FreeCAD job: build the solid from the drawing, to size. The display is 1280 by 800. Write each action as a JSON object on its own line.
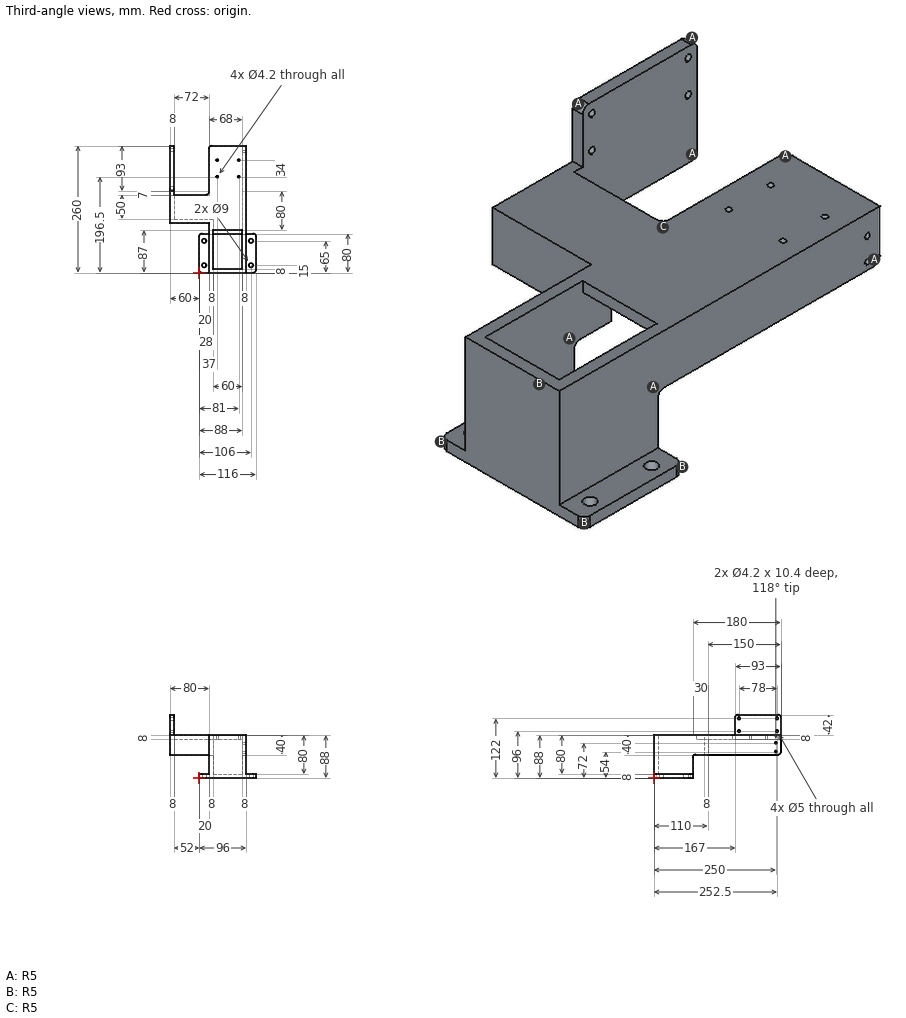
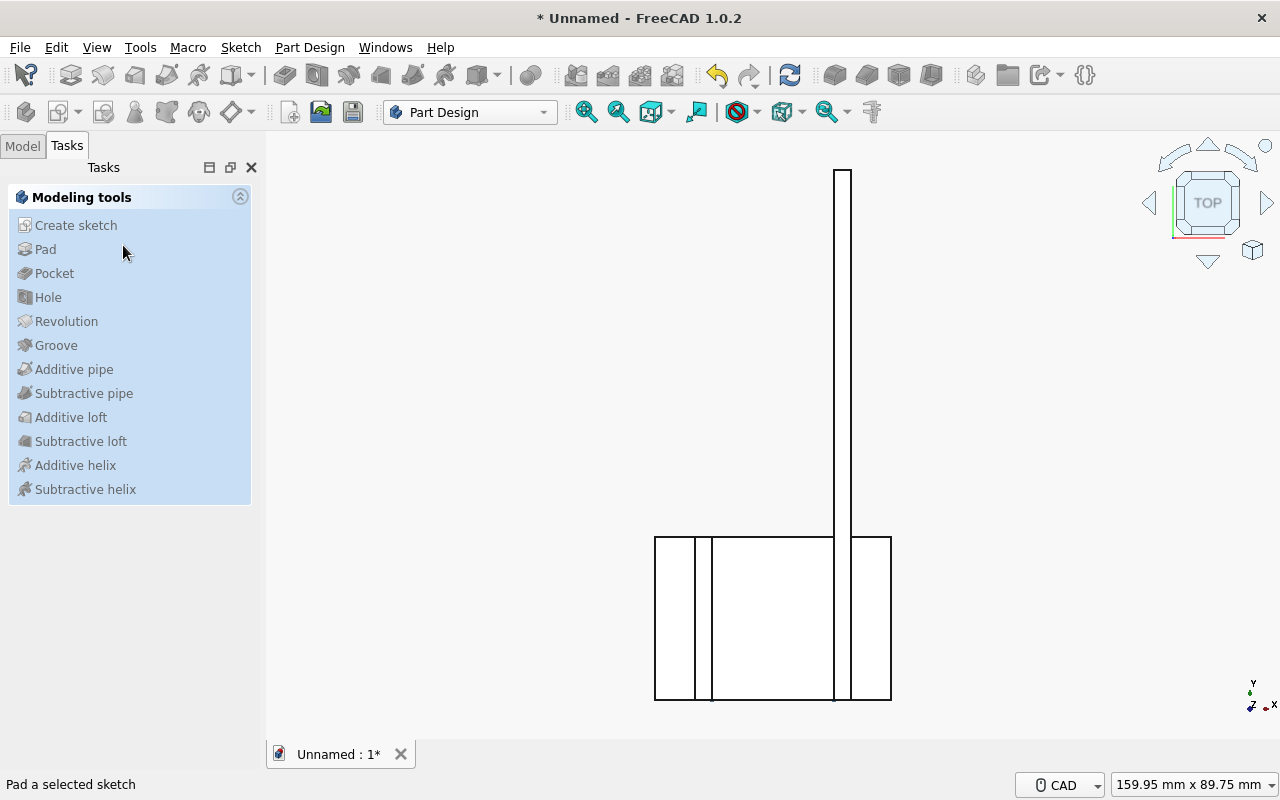
{"action": "left_click", "coordinate": [72, 76]}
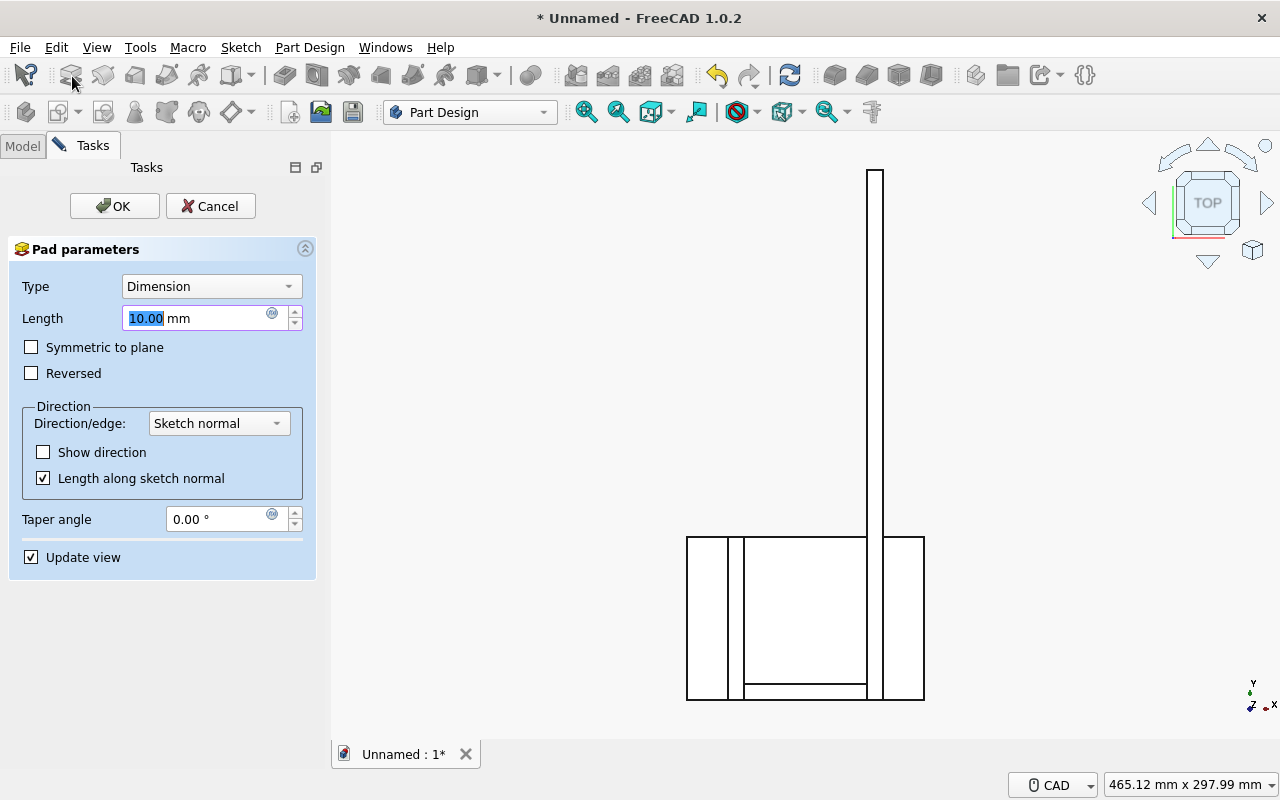
{"action": "type", "text": "80"}
{"action": "key", "text": "Tab"}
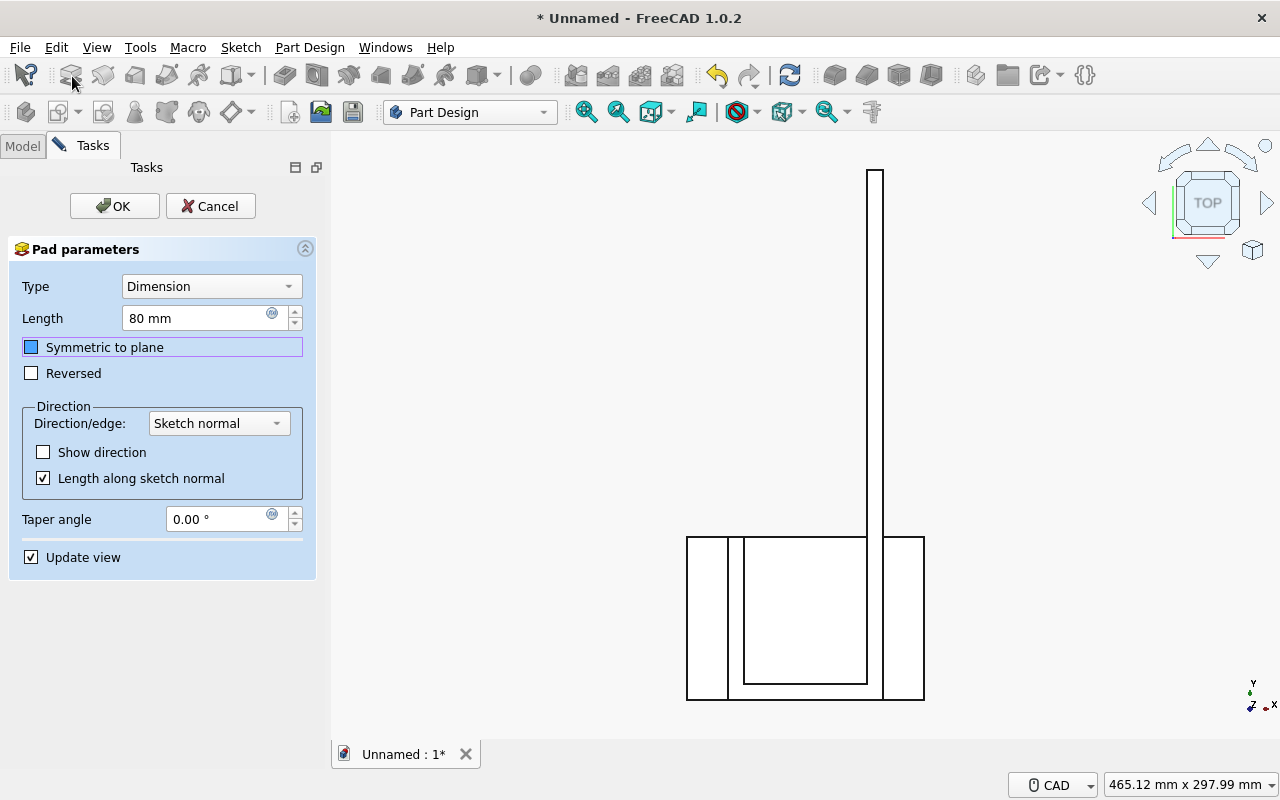
{"action": "left_click", "coordinate": [115, 206]}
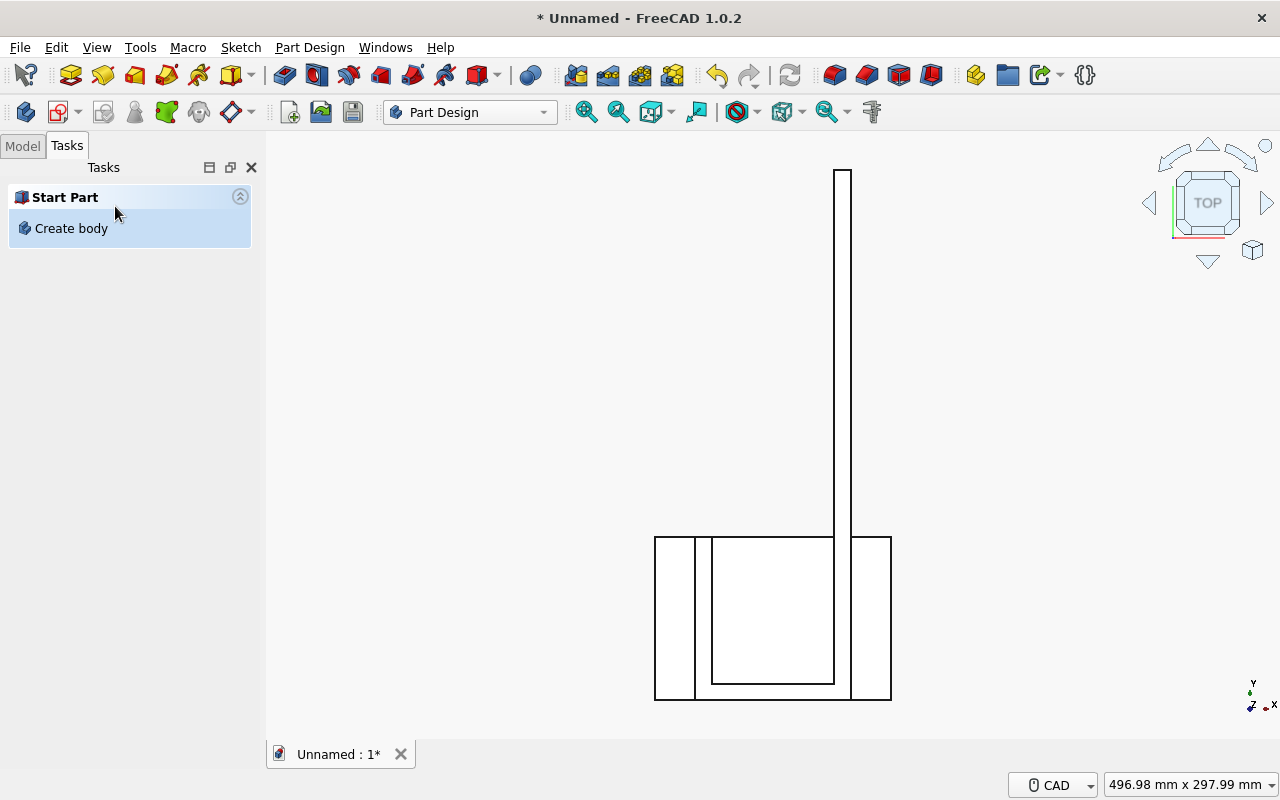
{"action": "key", "text": "4"}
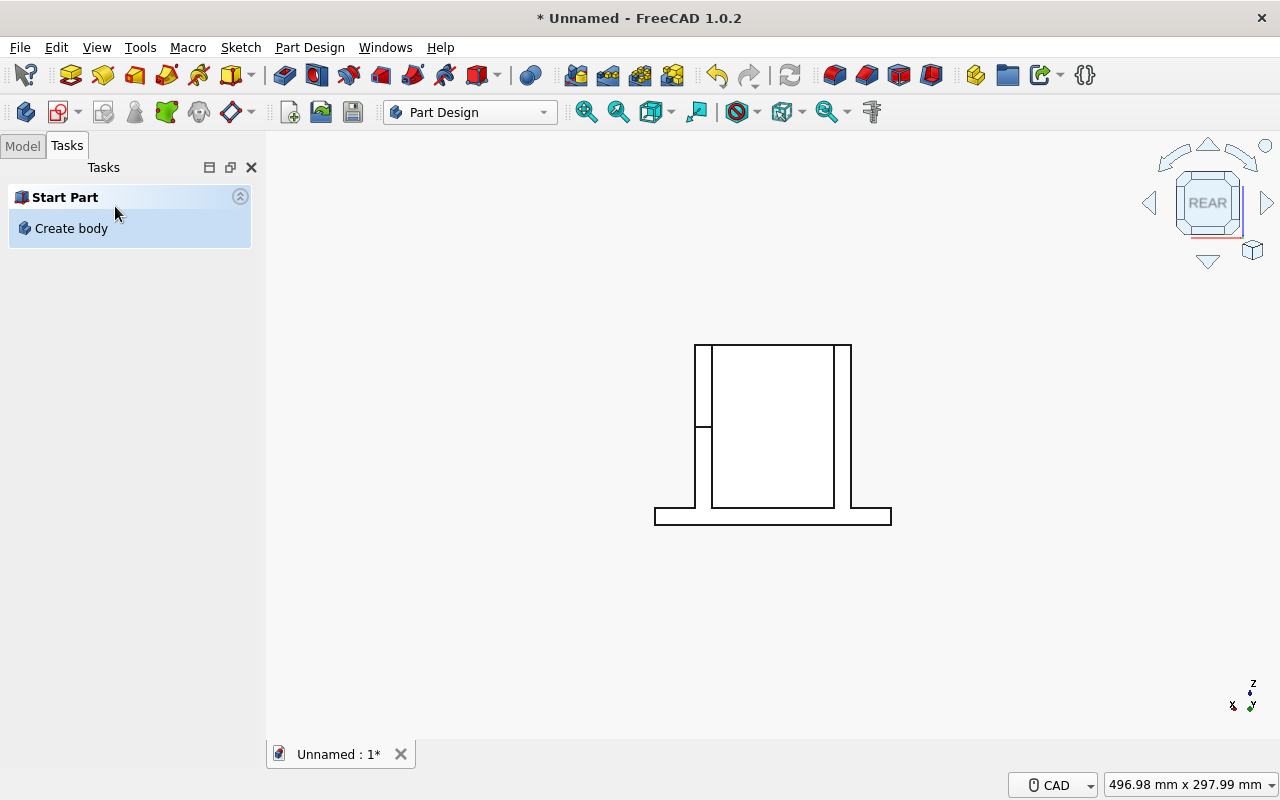
{"action": "left_click", "coordinate": [588, 112]}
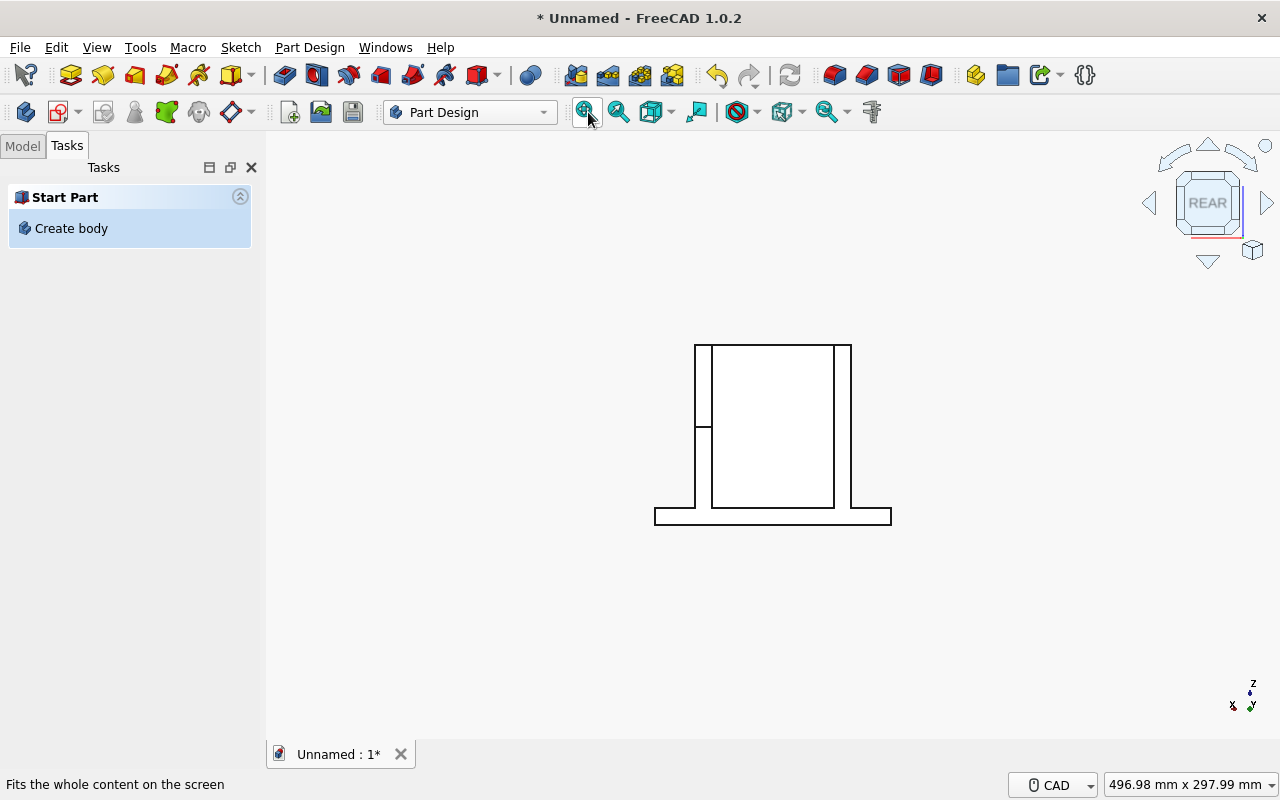
{"action": "key", "text": "2"}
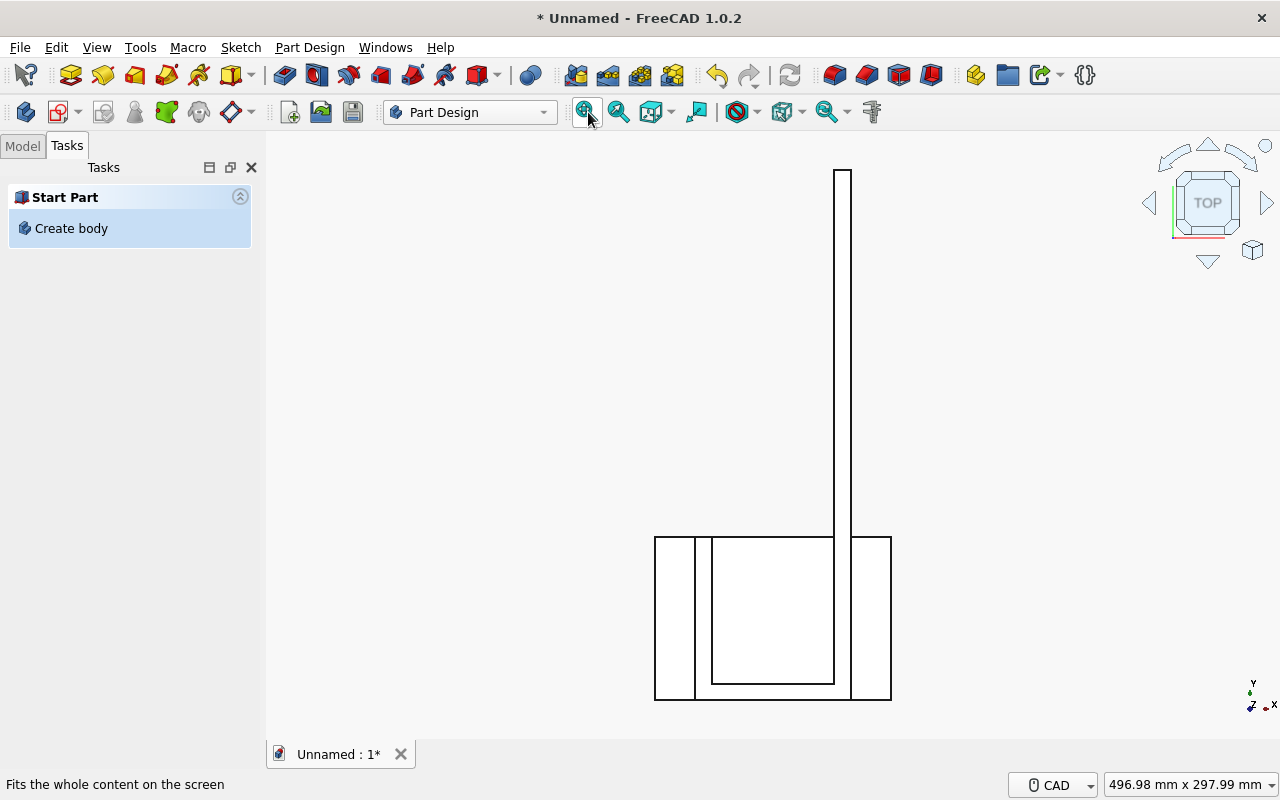
{"action": "key", "text": "3"}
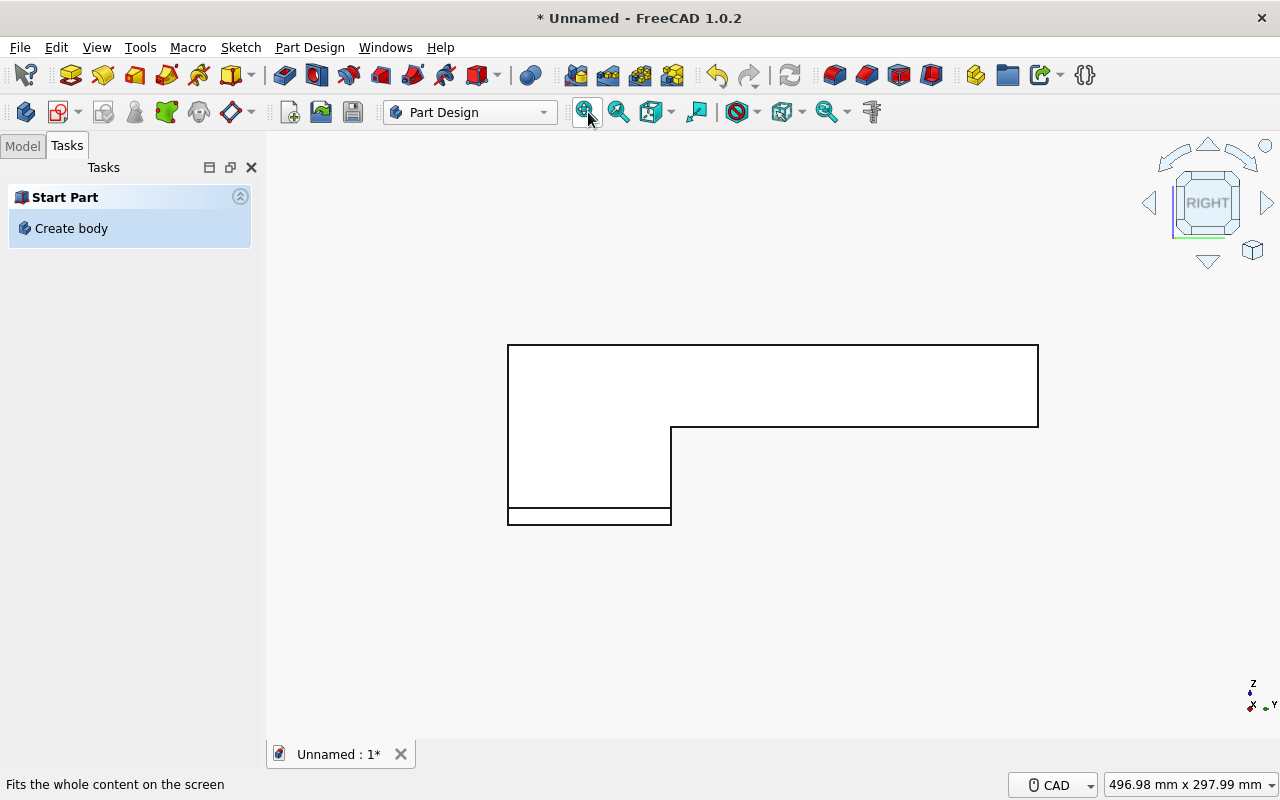
{"action": "left_click", "coordinate": [23, 145]}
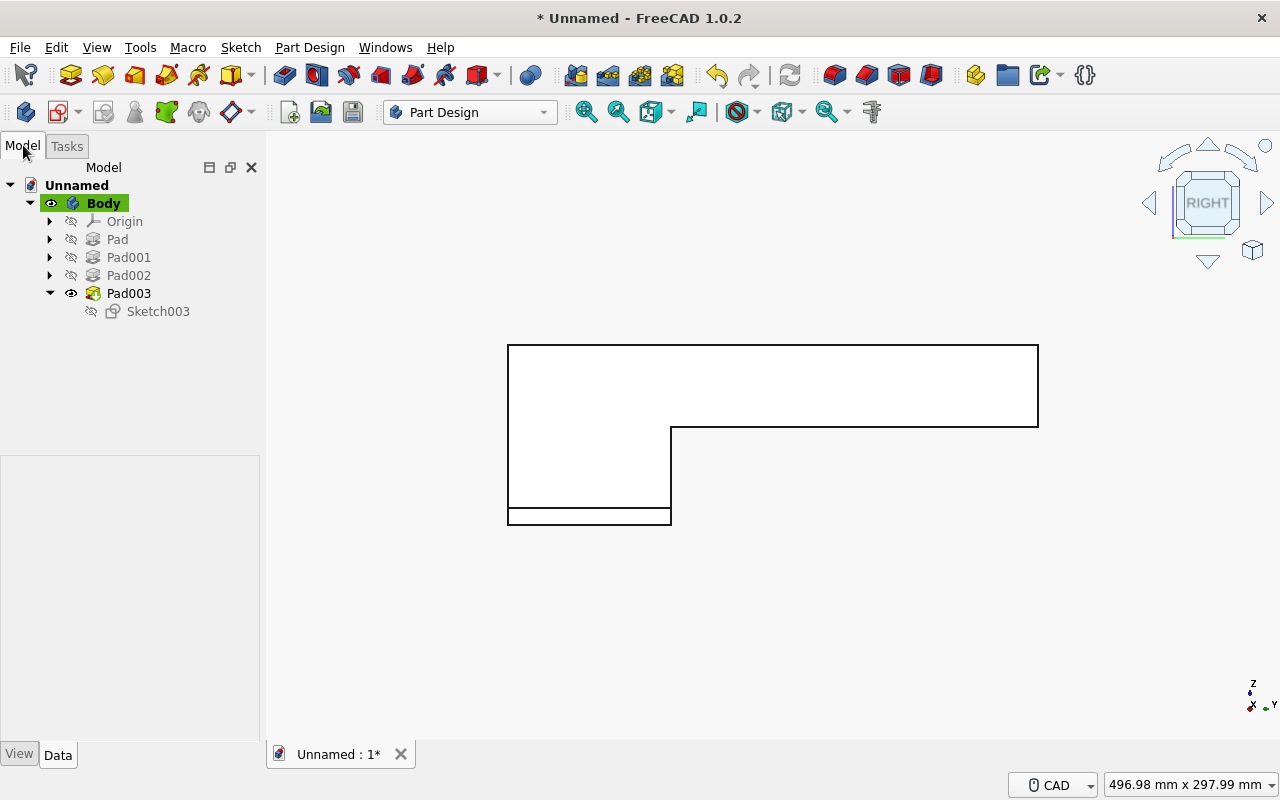
{"action": "left_click", "coordinate": [50, 221]}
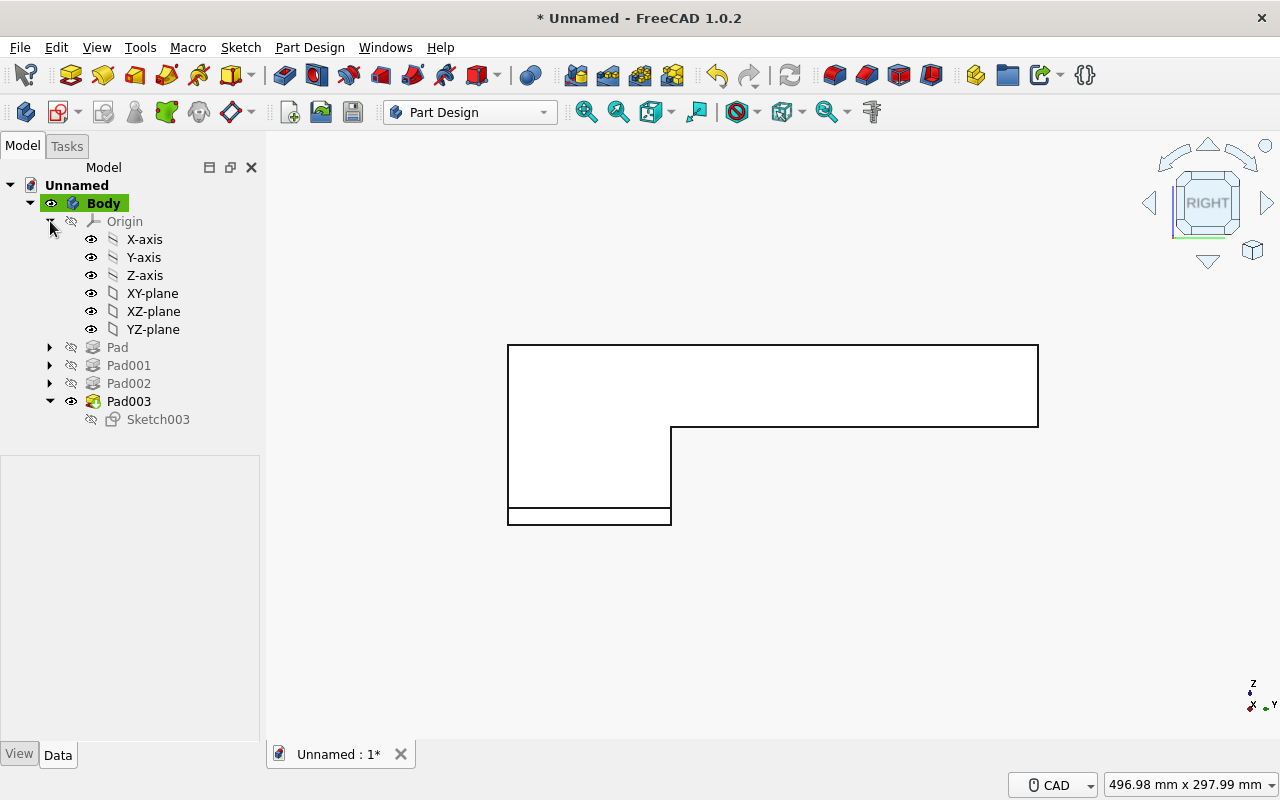
{"action": "left_click", "coordinate": [136, 311]}